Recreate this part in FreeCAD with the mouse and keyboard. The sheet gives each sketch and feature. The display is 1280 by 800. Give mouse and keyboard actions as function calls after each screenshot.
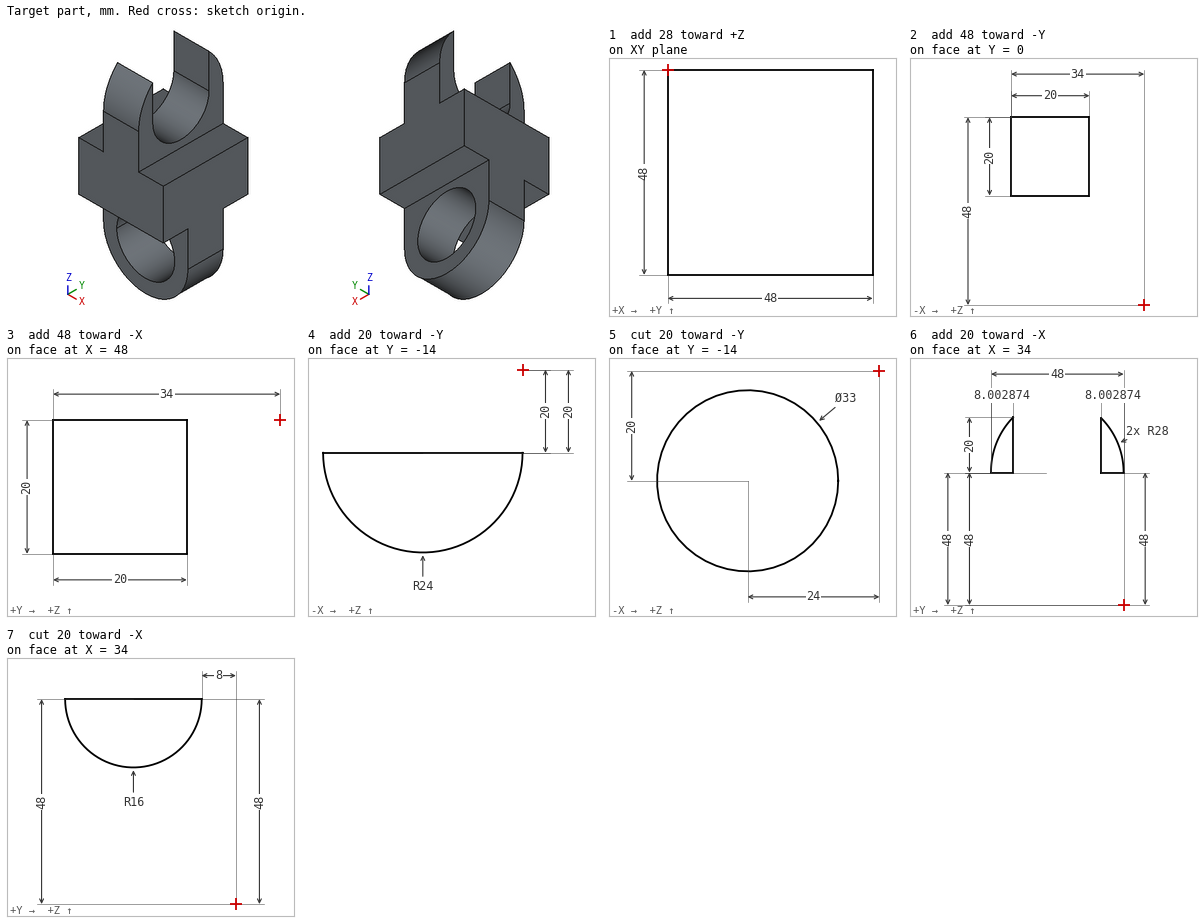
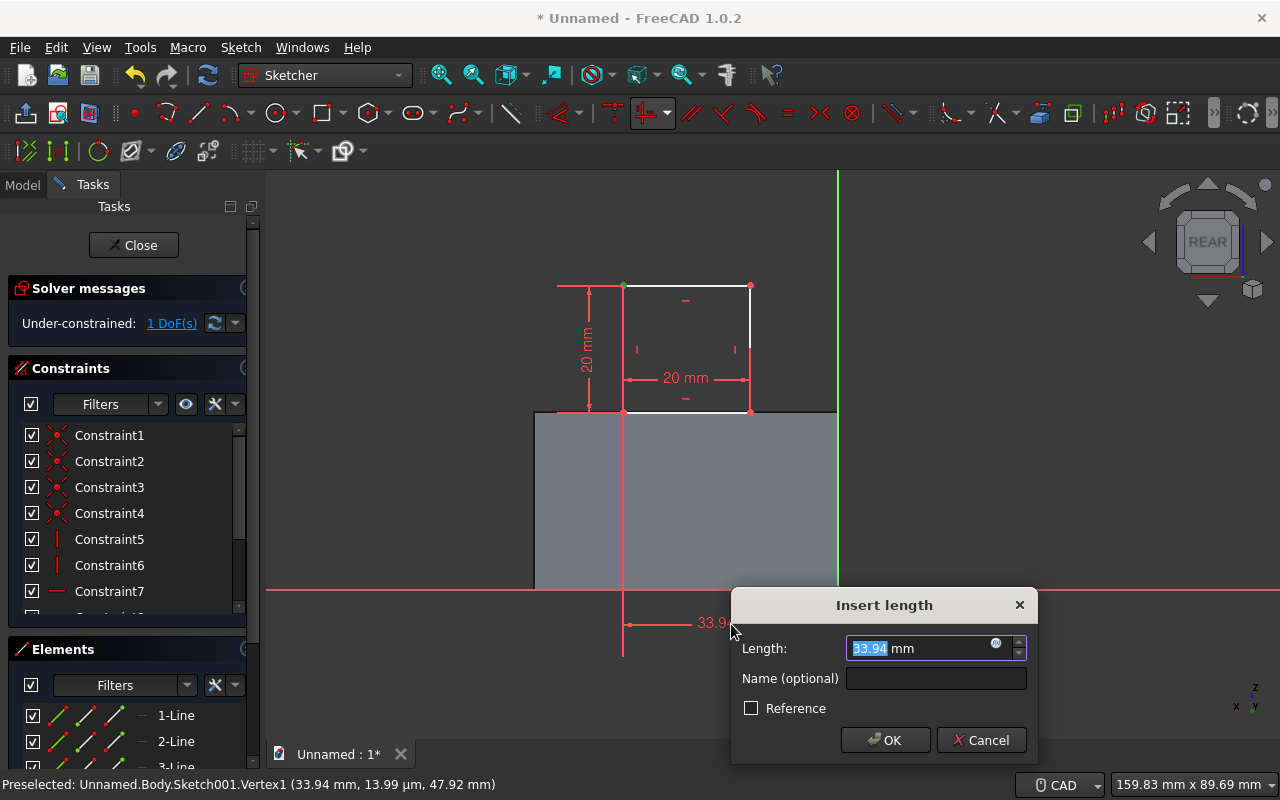
text(34)
key(Return)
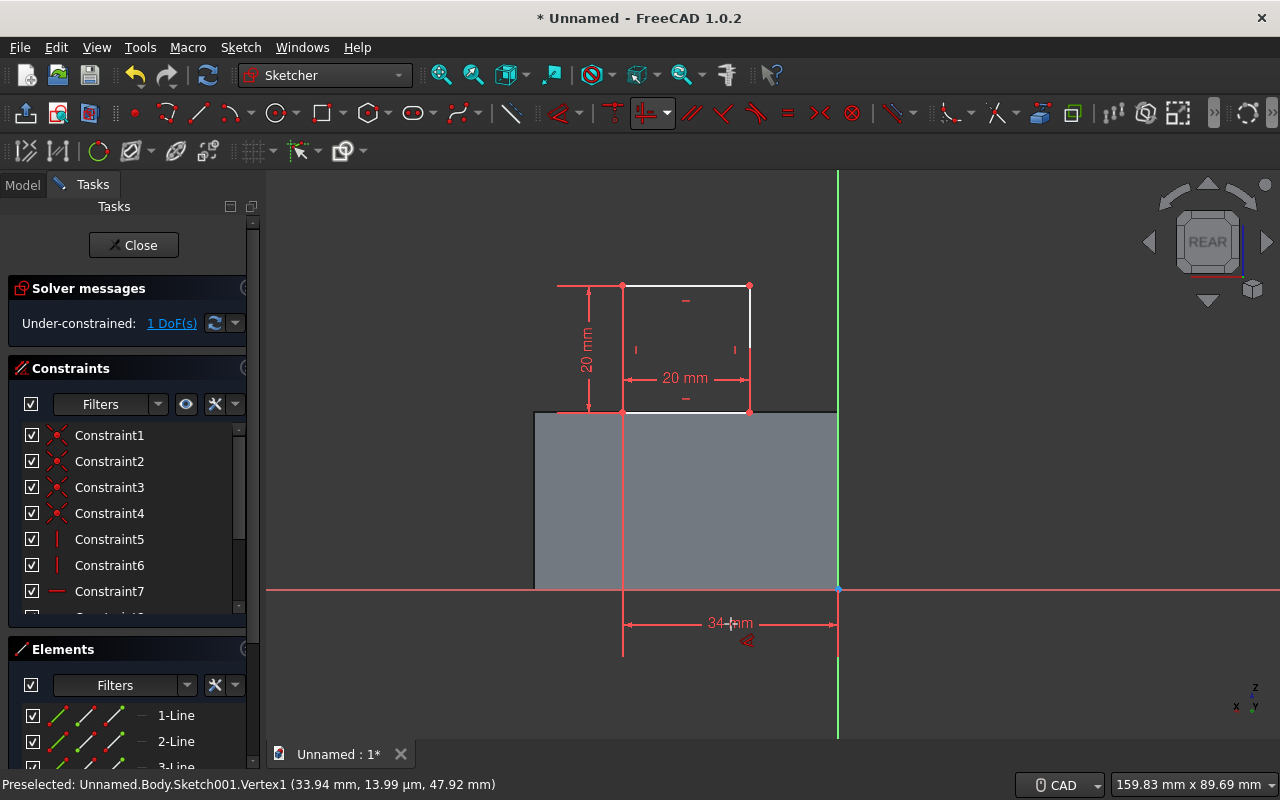
click(623, 286)
click(872, 438)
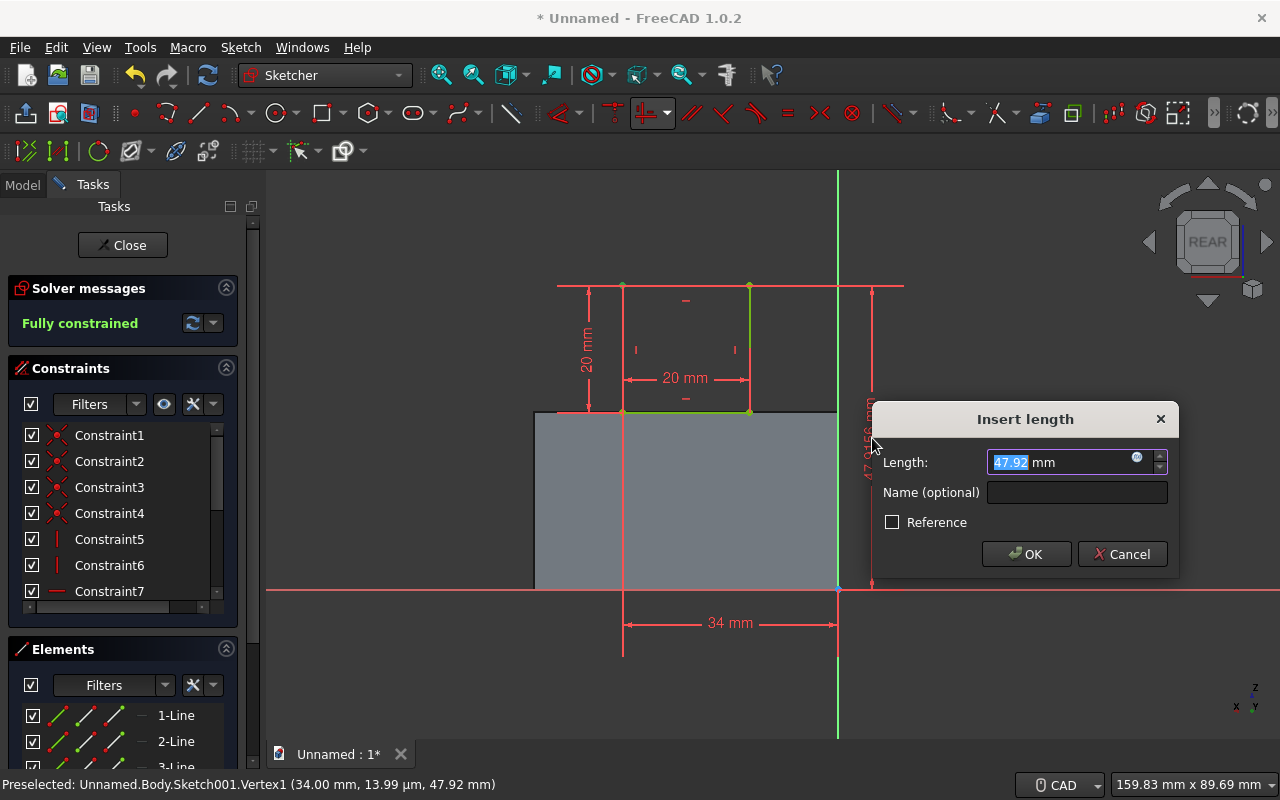
text(48)
key(Return)
key(Escape)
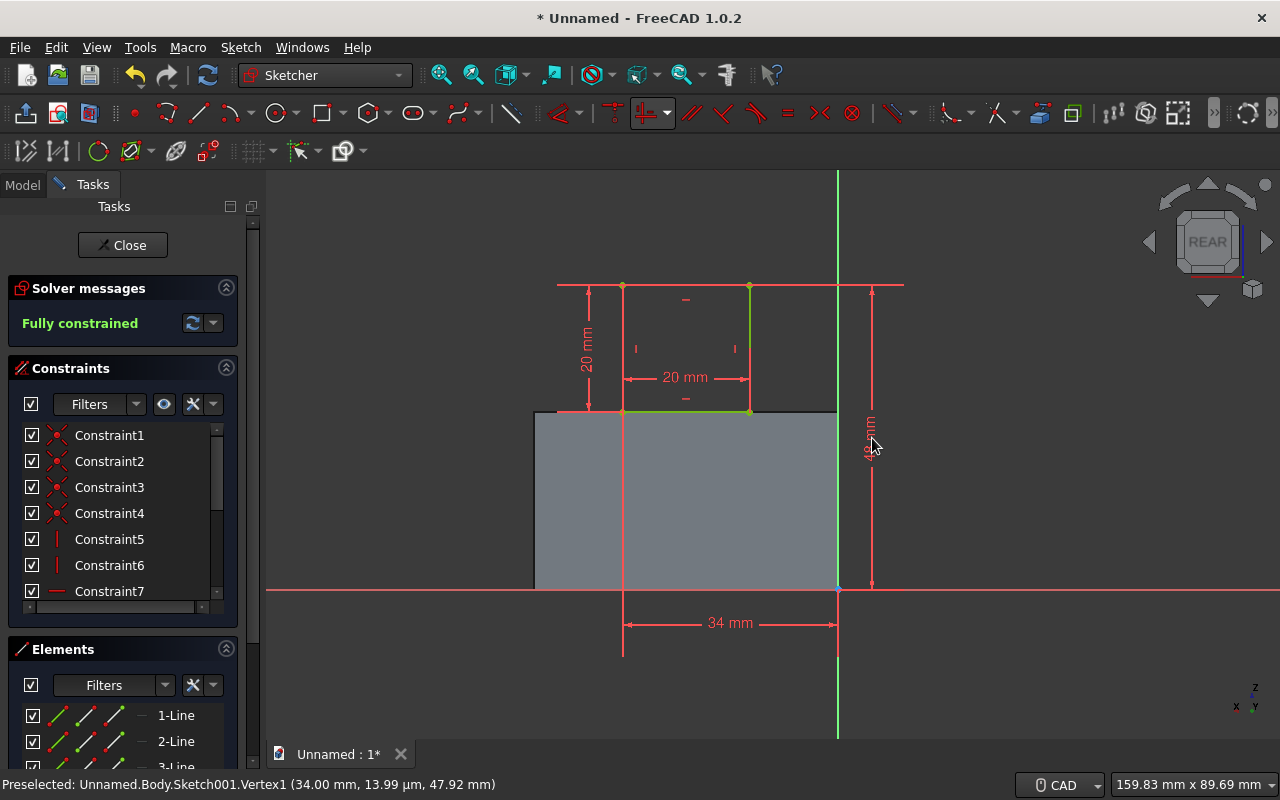
click(123, 245)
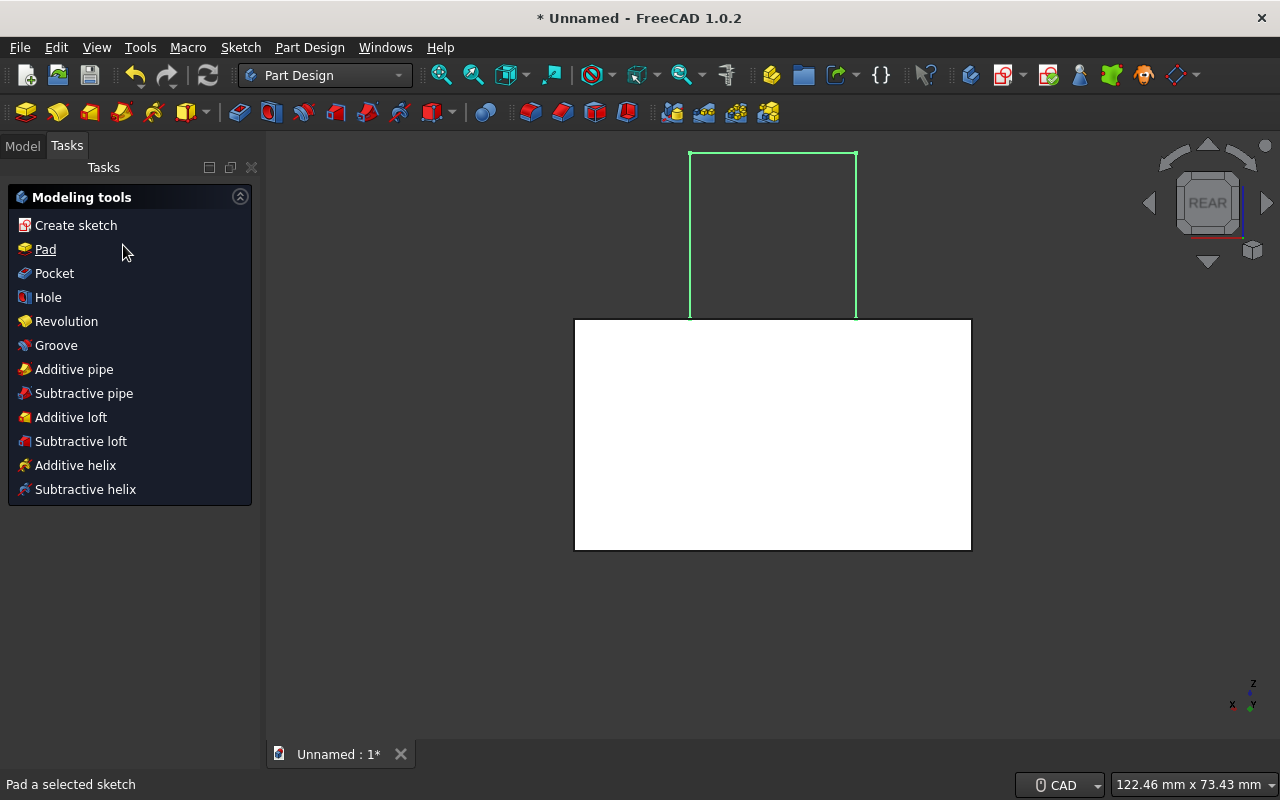
click(26, 112)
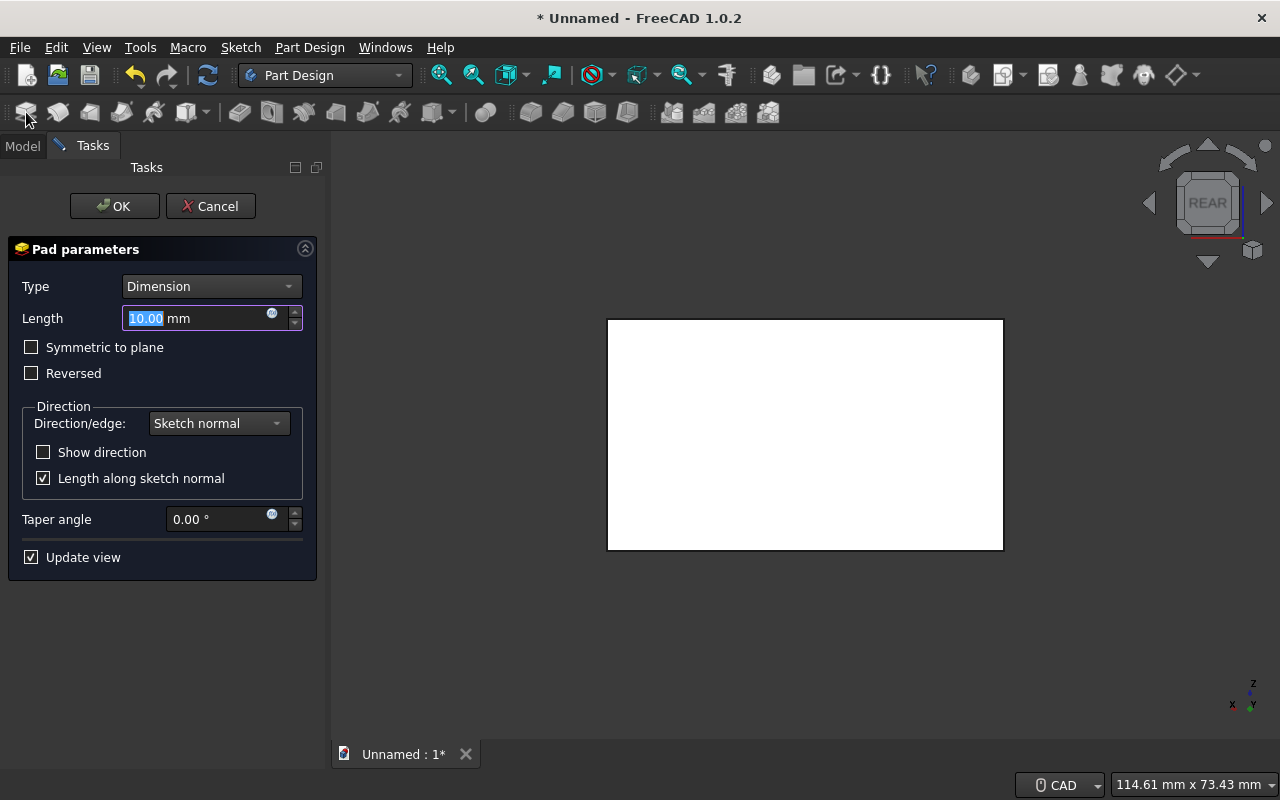
text(48)
key(Tab)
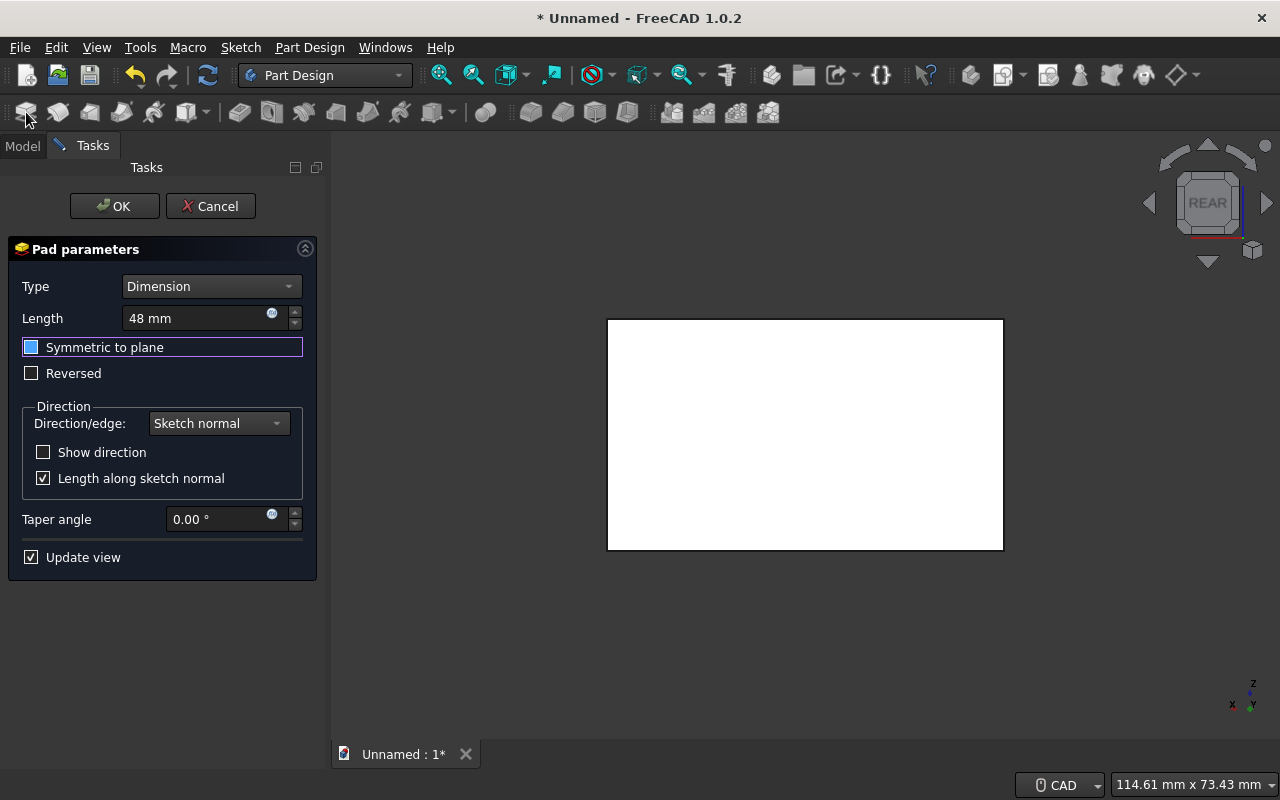
click(30, 373)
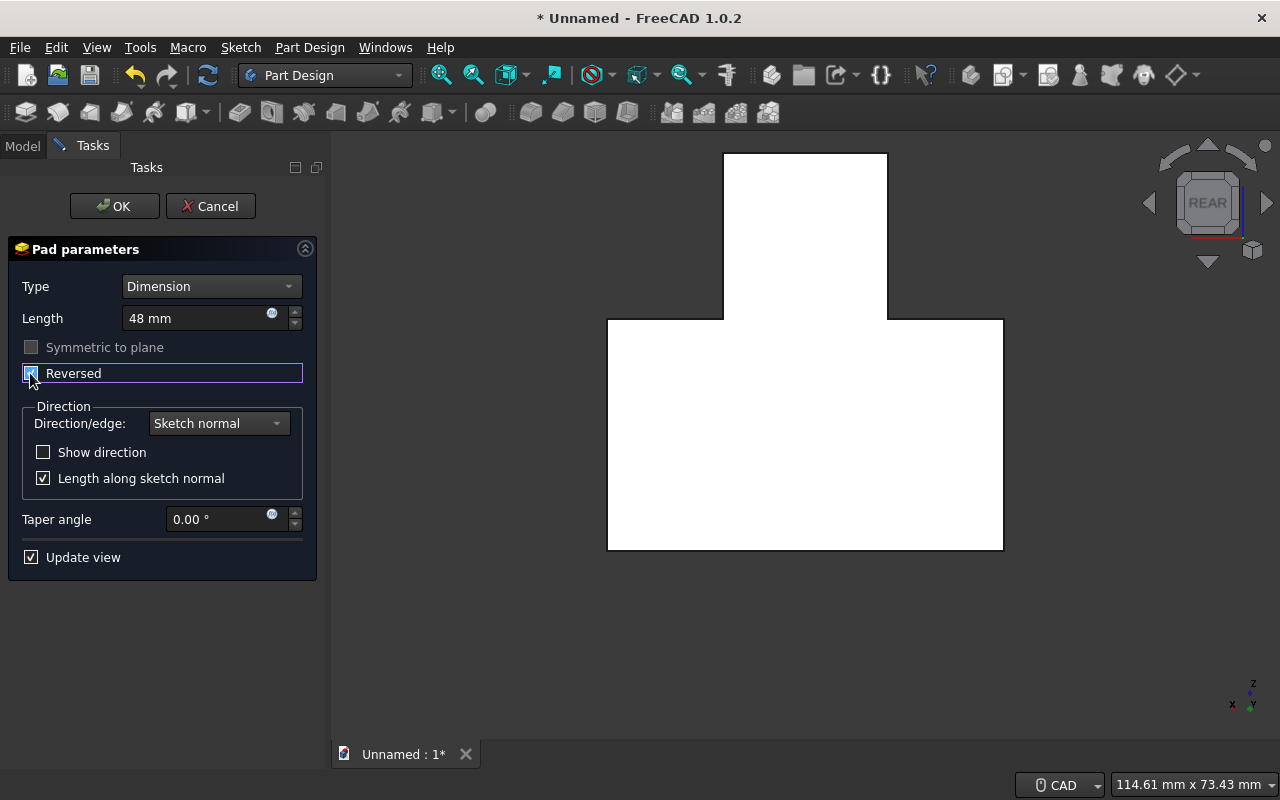
click(115, 206)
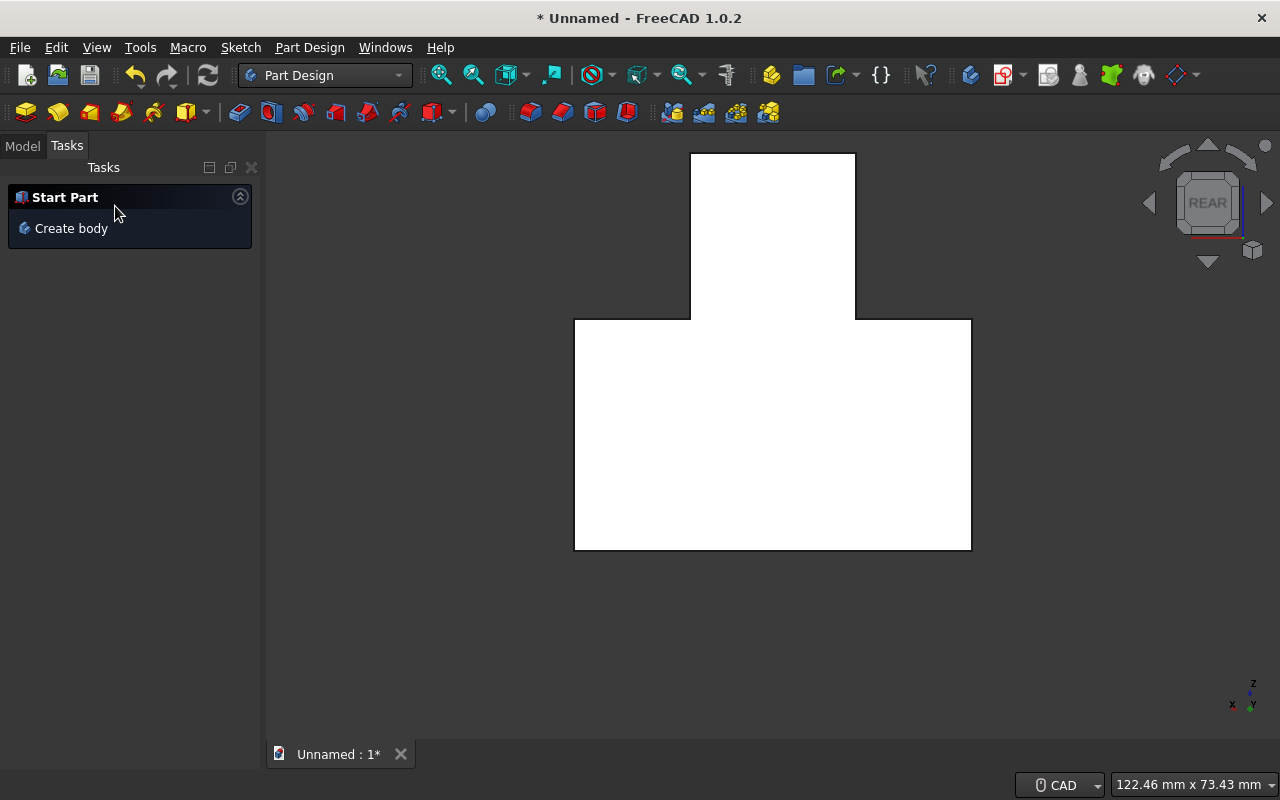
key(0)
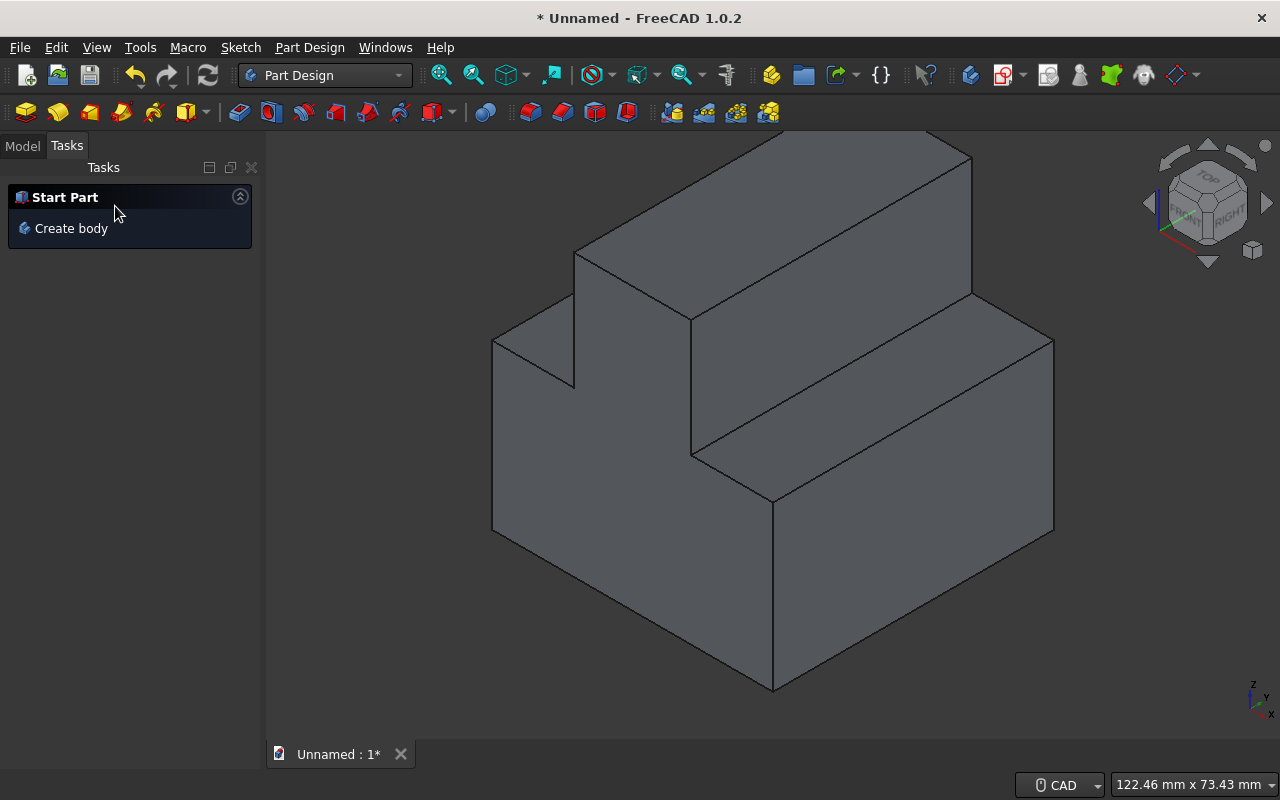
key(v)
key(f)